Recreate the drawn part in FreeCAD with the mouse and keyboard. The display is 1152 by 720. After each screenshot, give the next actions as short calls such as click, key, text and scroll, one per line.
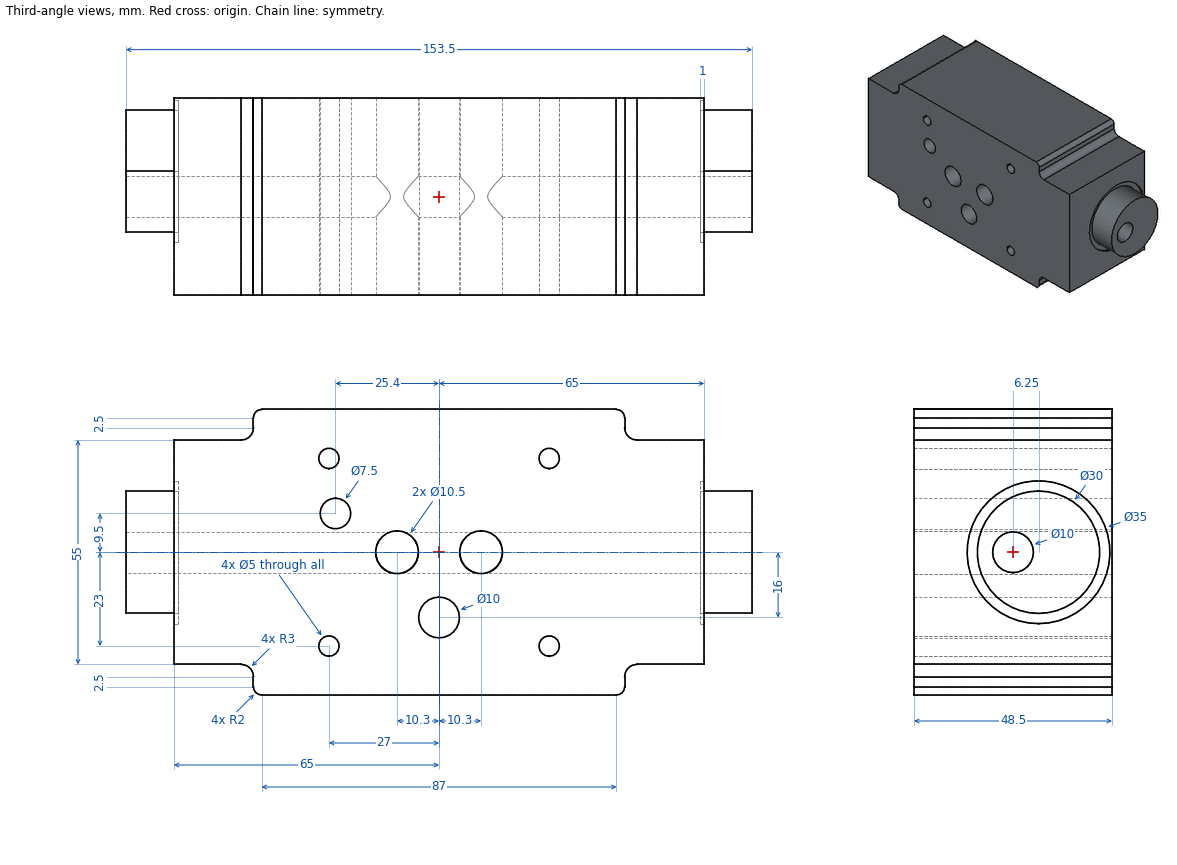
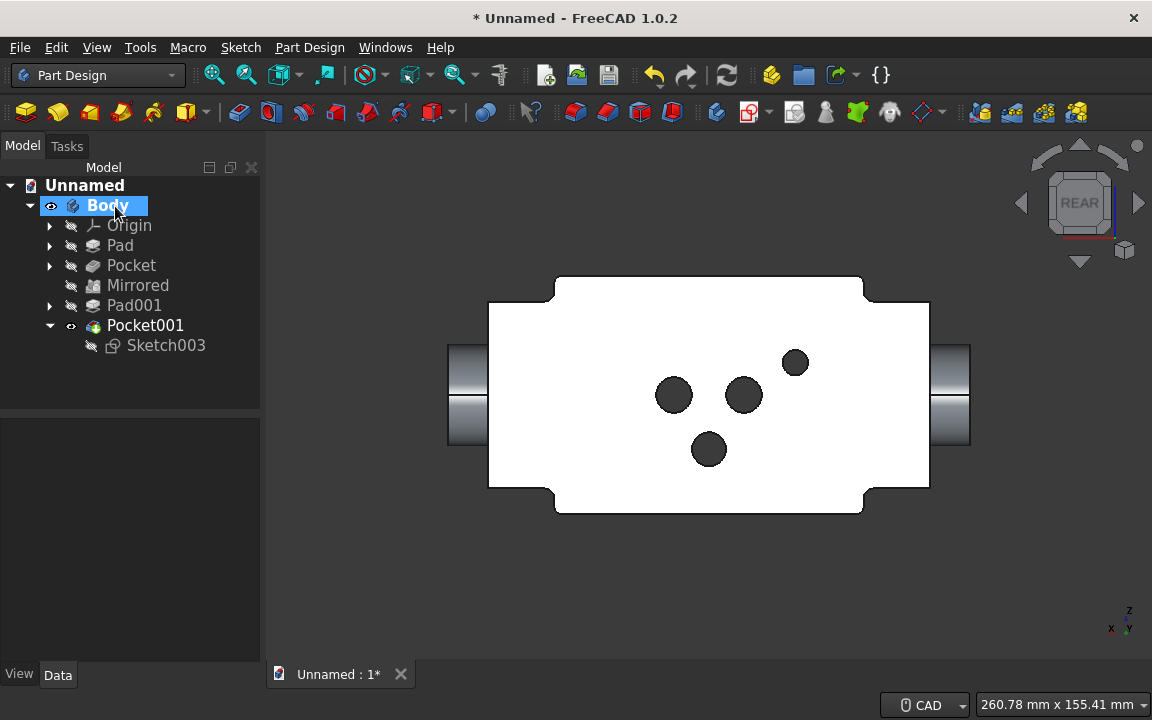
click(583, 394)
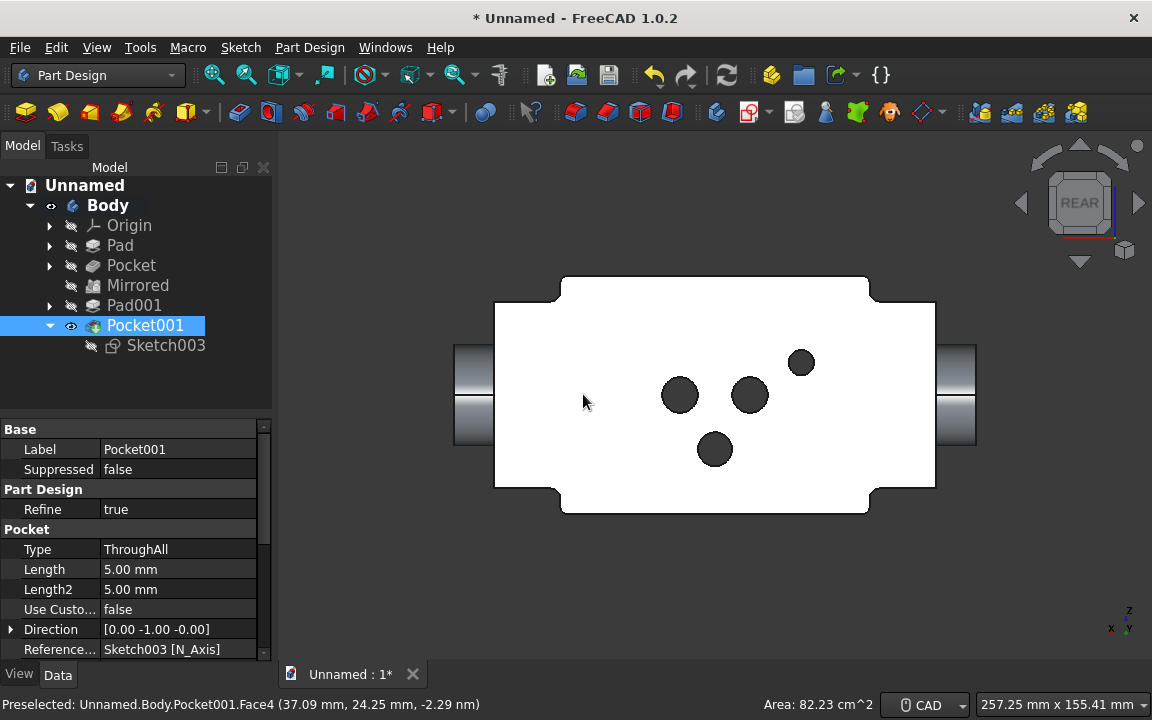
click(750, 112)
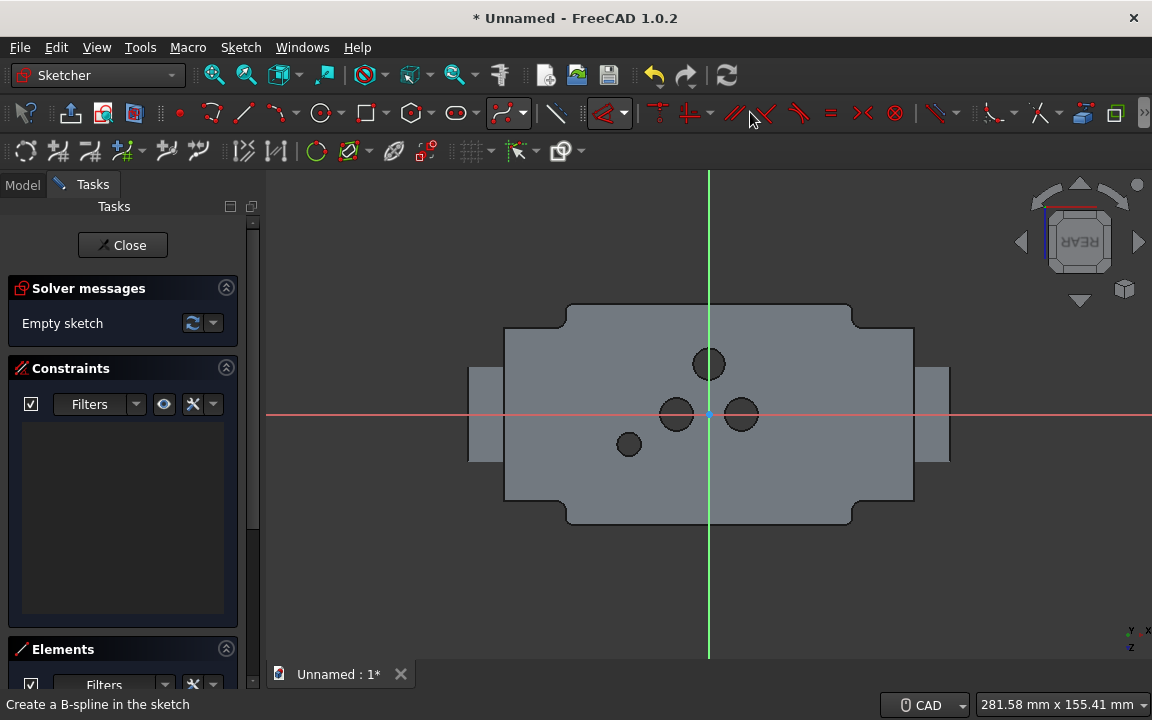
scroll(792, 414, up, 3)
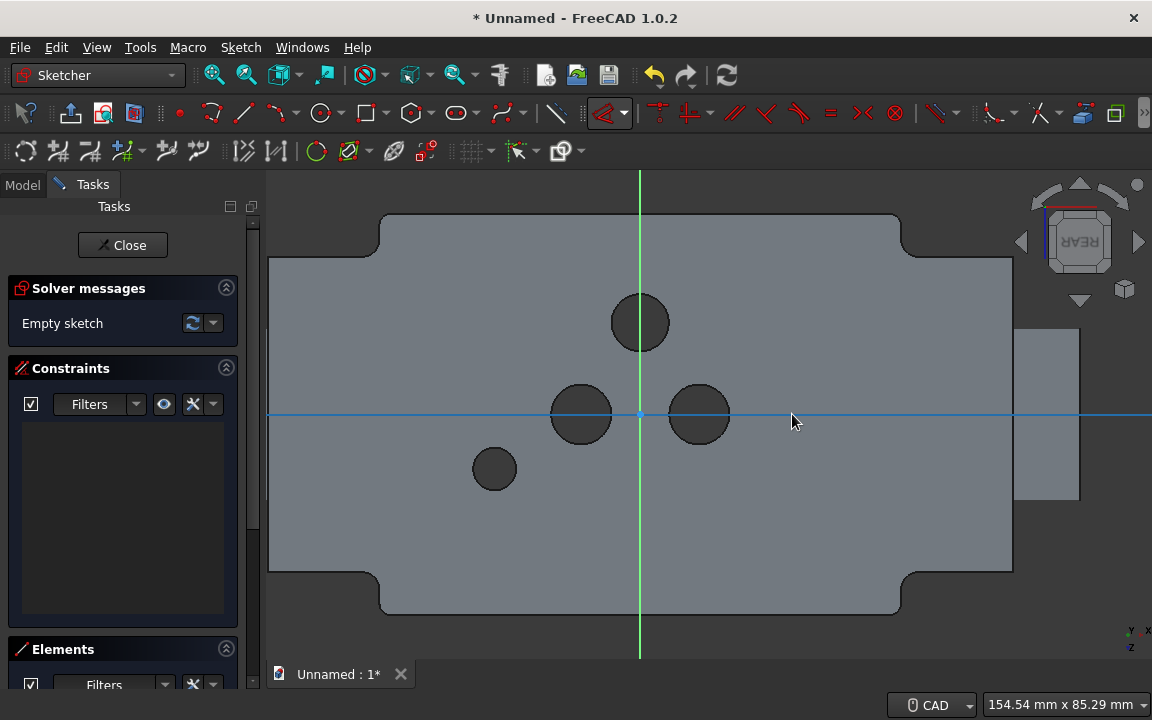
click(322, 114)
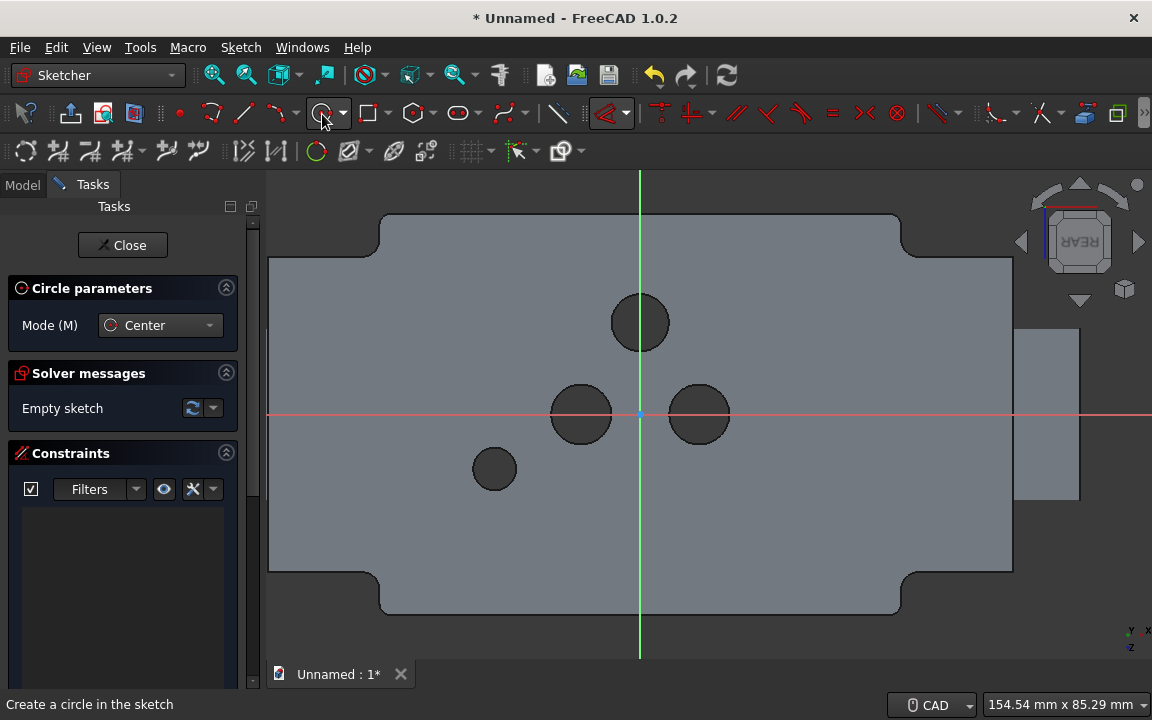
scroll(485, 283, up, 3)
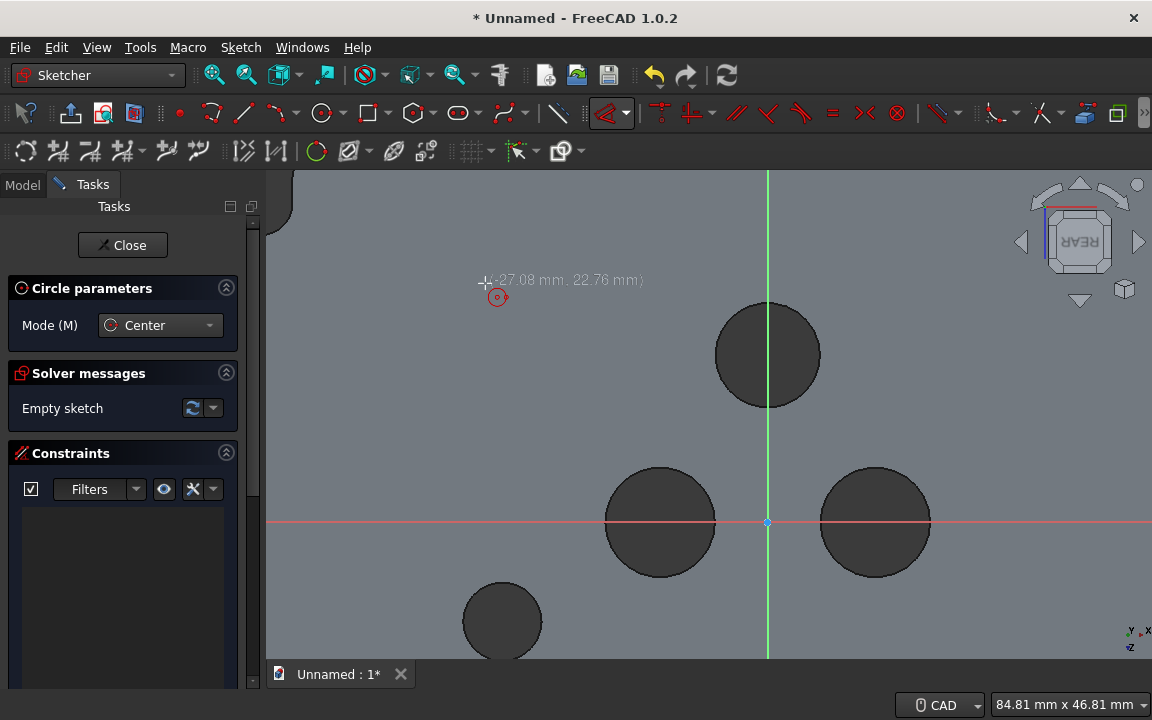
click(486, 282)
move(504, 264)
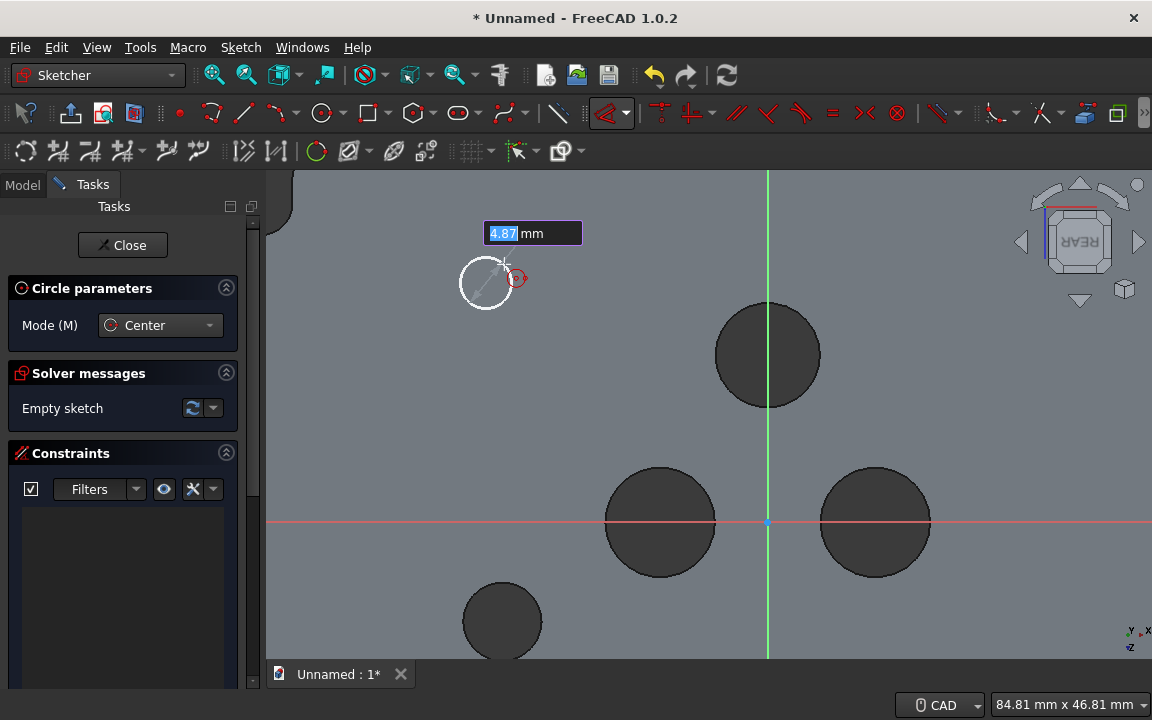
text(5)
key(Return)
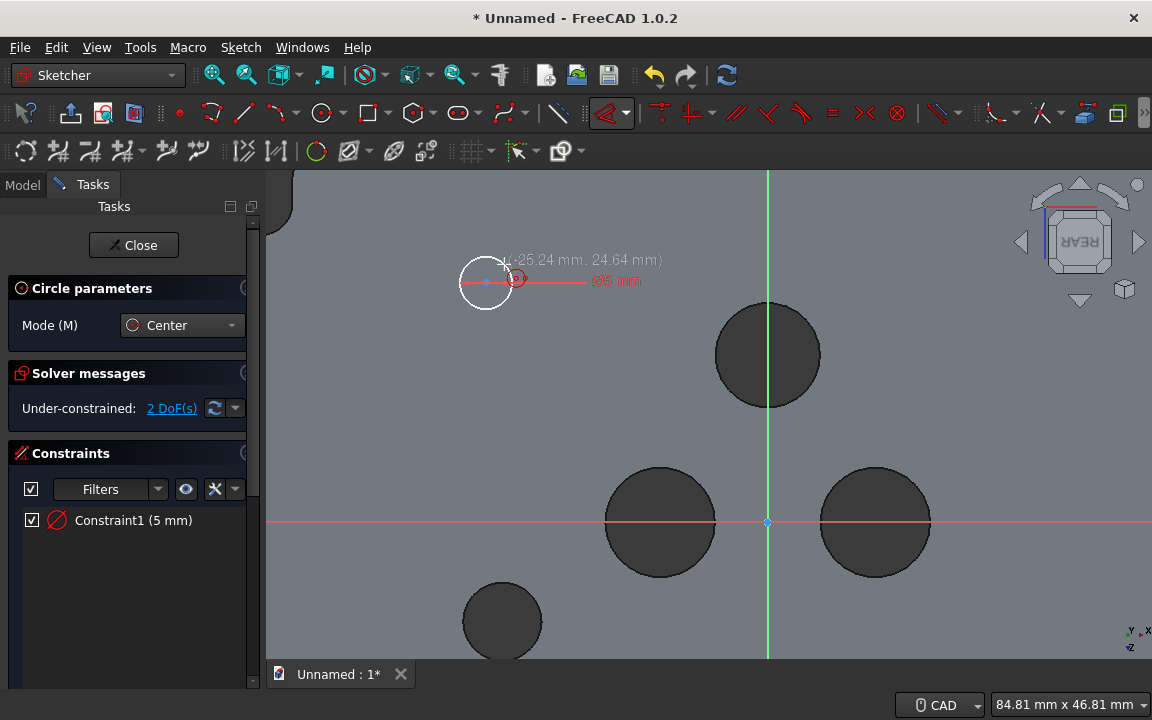
scroll(486, 283, down, 3)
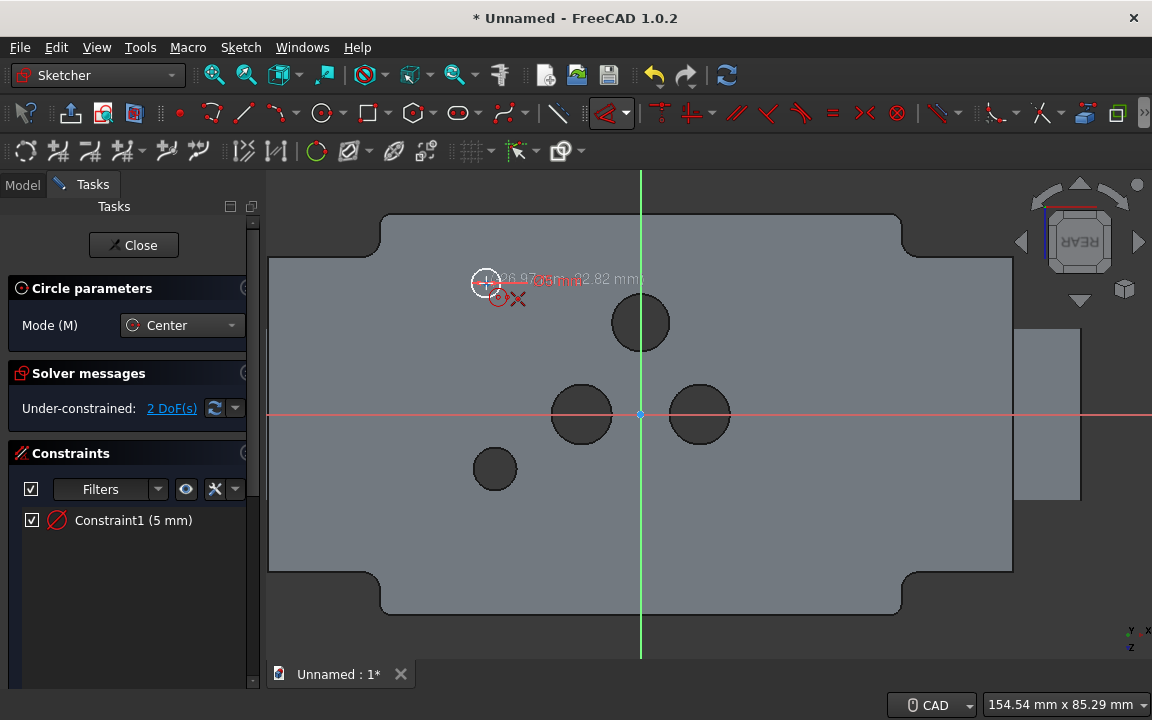
scroll(796, 283, up, 3)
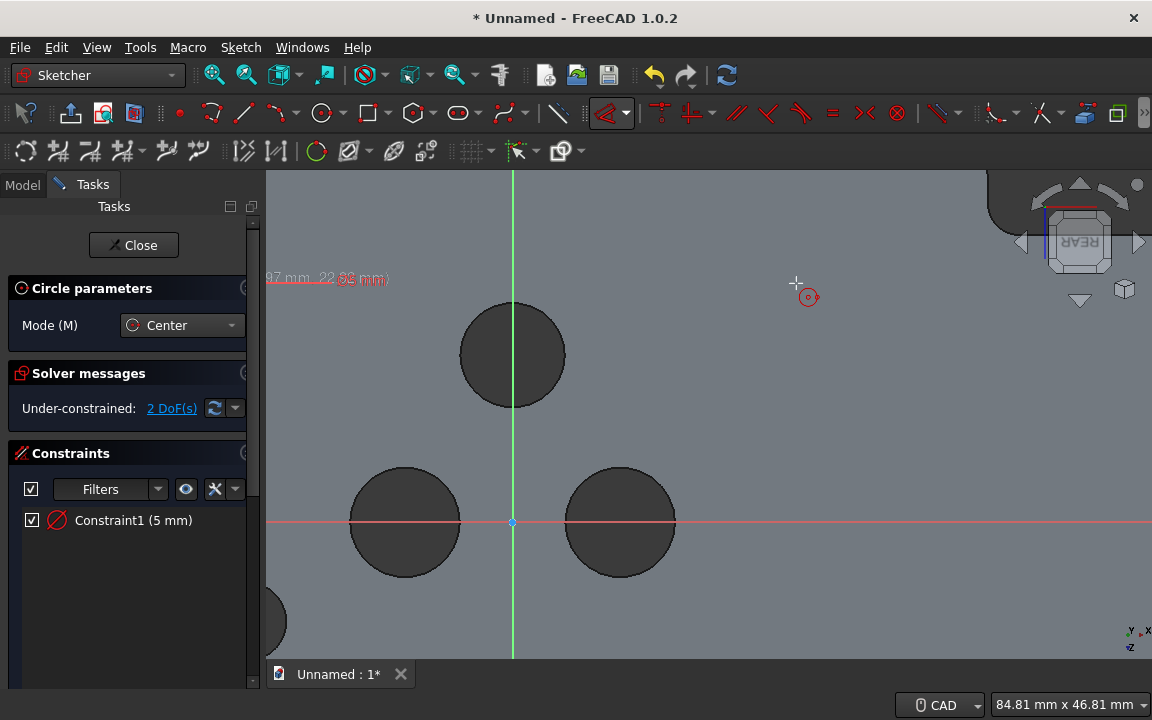
click(795, 282)
move(813, 264)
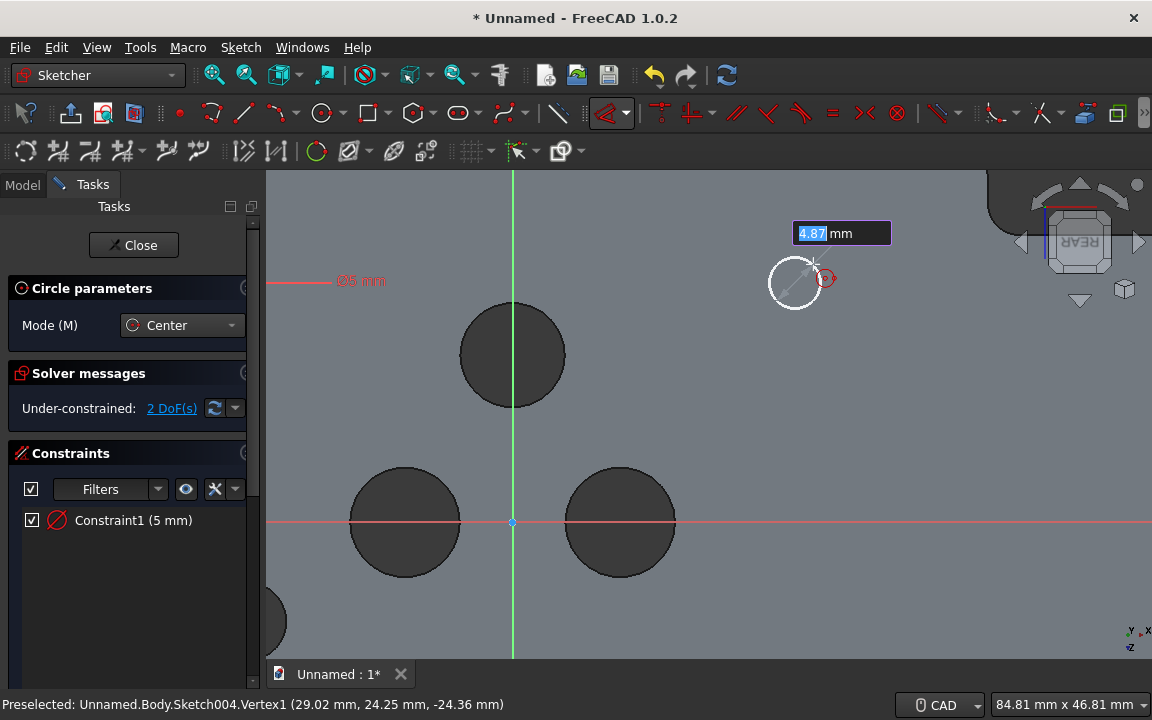
text(5)
key(Return)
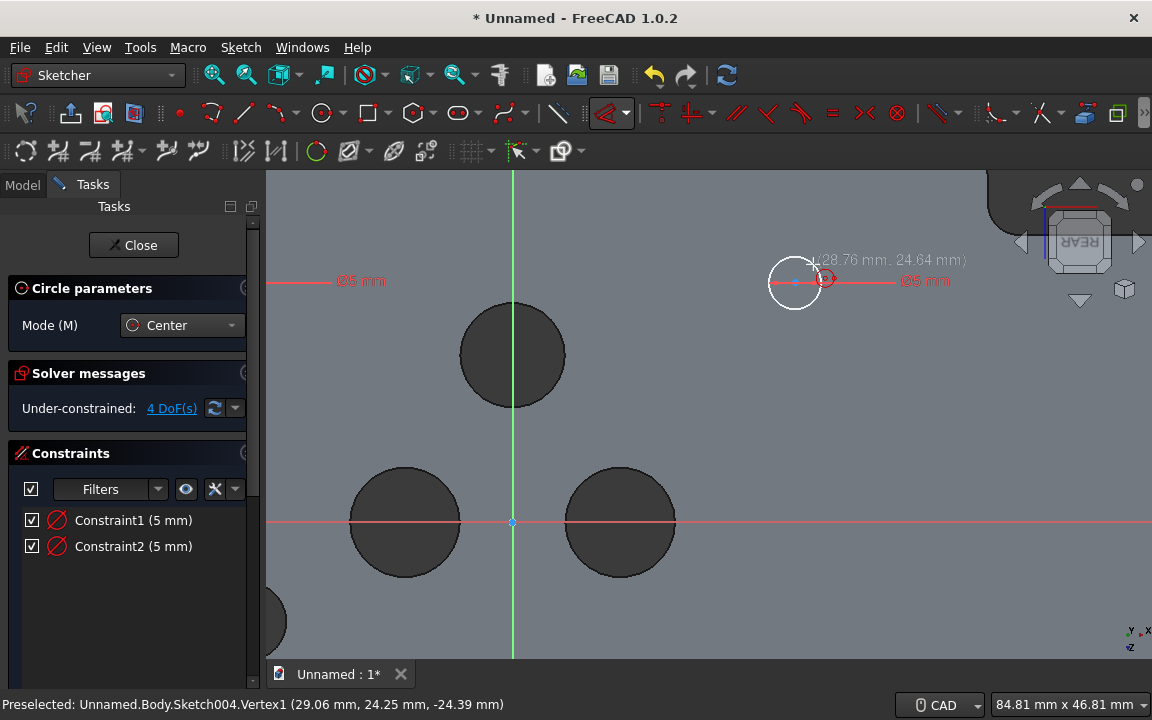
scroll(796, 283, down, 3)